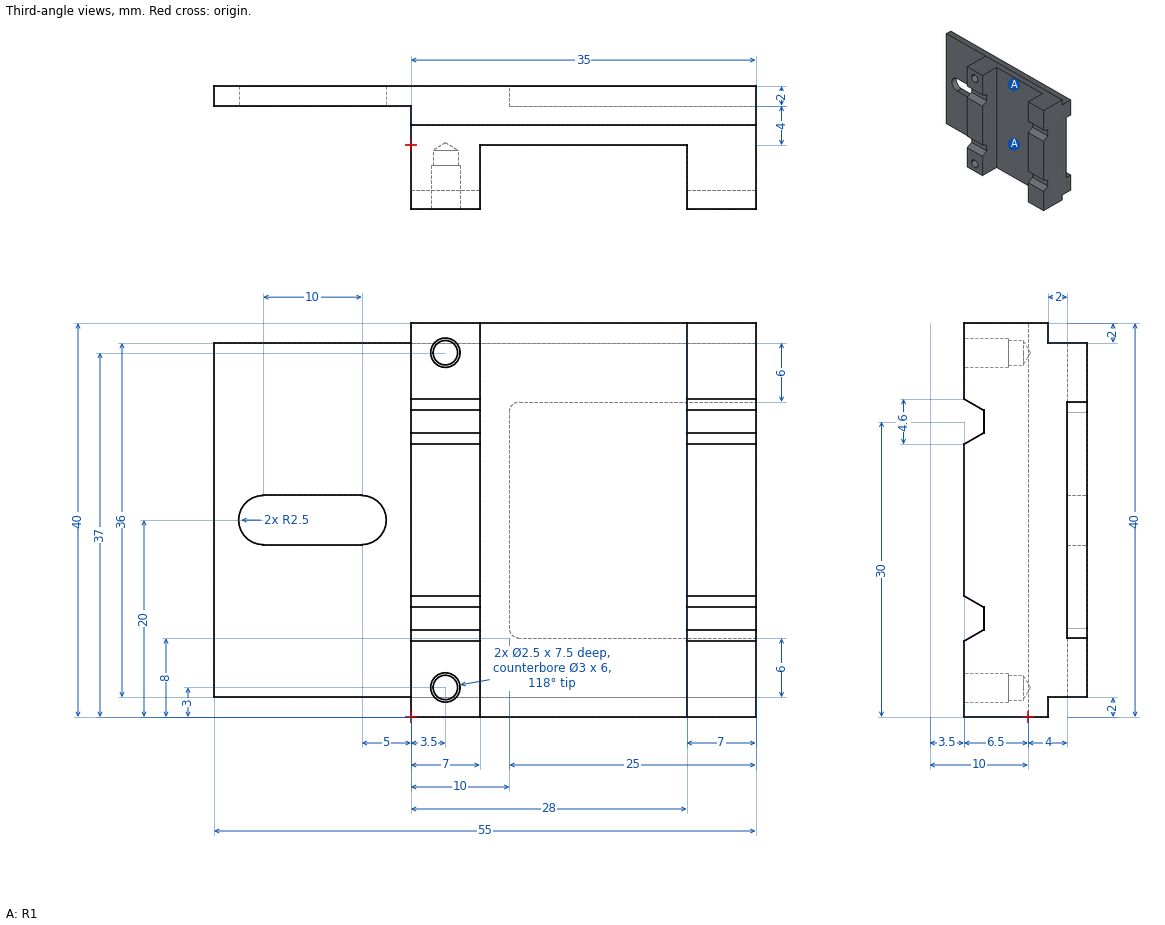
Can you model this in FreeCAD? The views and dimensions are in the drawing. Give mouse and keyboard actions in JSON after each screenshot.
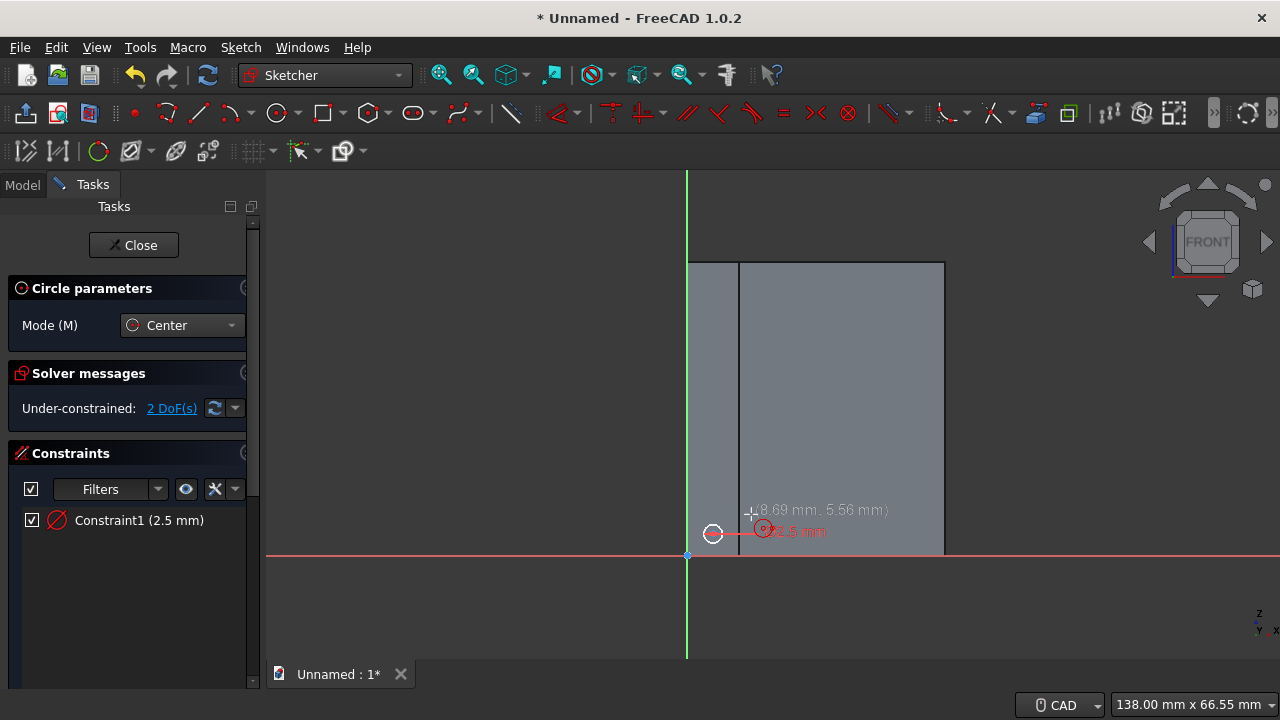
{"action": "scroll", "coordinate": [713, 284], "scroll_direction": "up", "scroll_amount": 5}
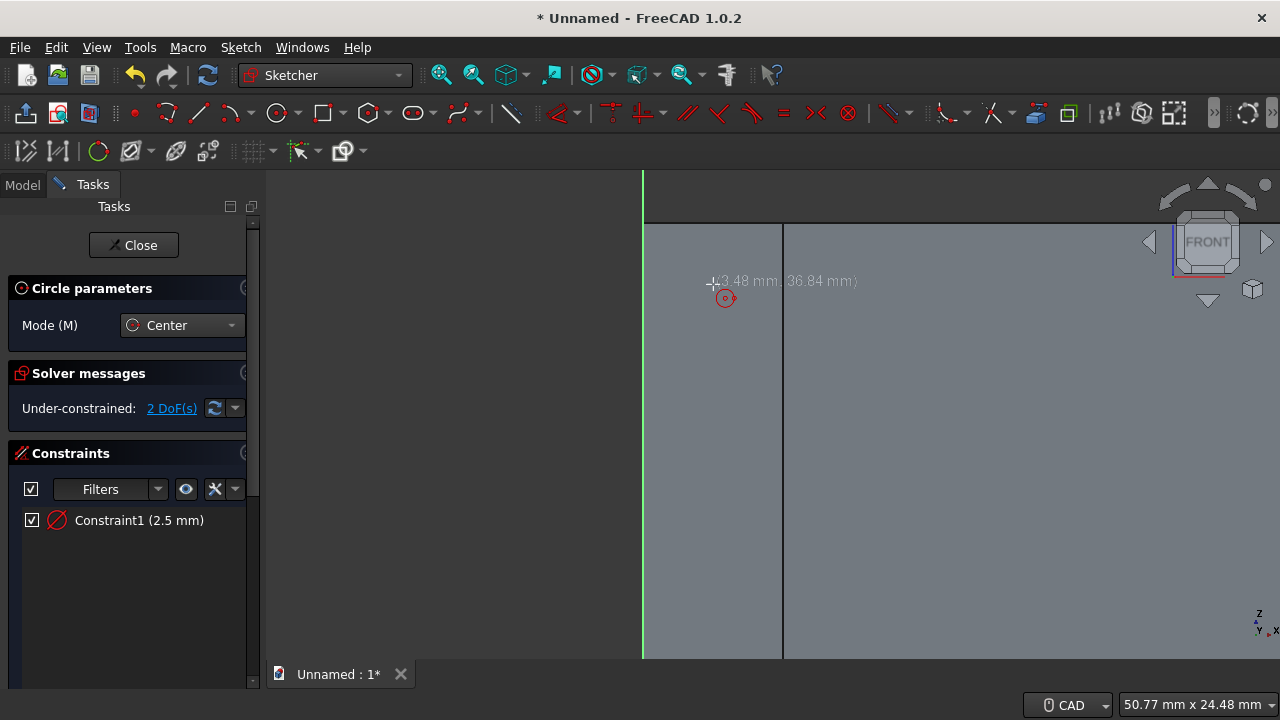
{"action": "left_click", "coordinate": [713, 283]}
{"action": "mouse_move", "coordinate": [730, 265]}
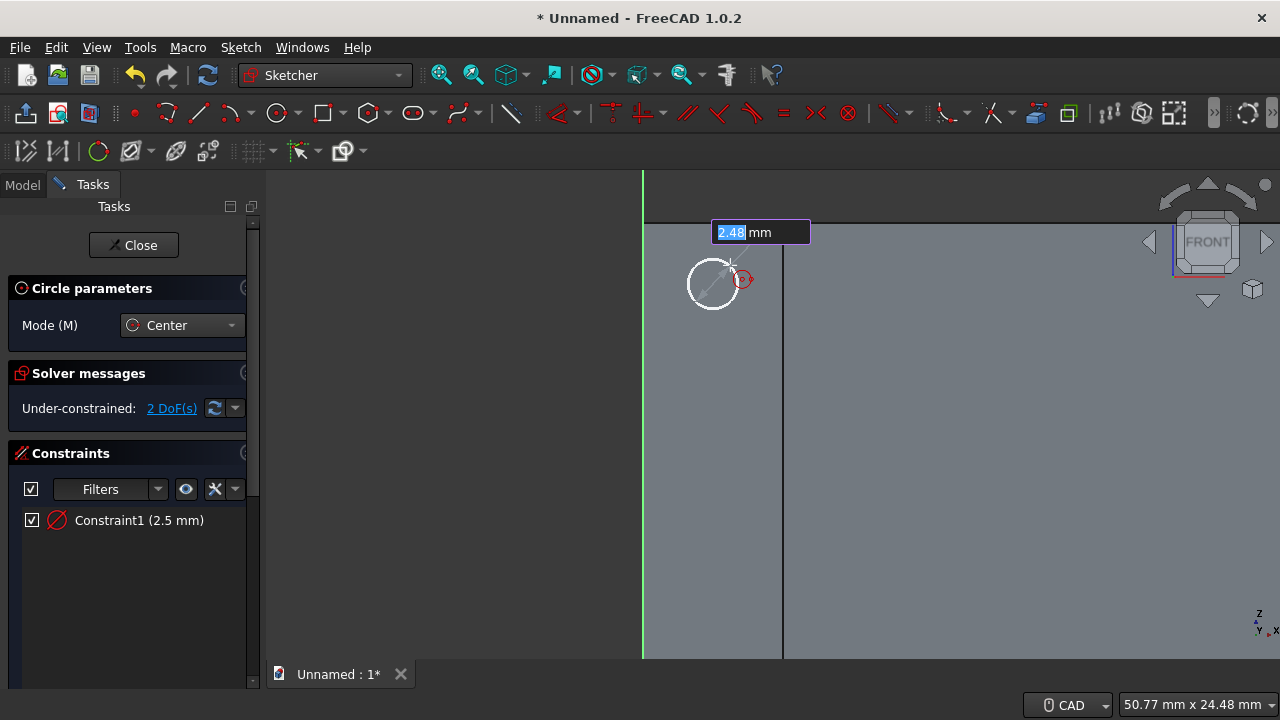
{"action": "type", "text": "2.5"}
{"action": "key", "text": "Return"}
{"action": "key", "text": "Escape"}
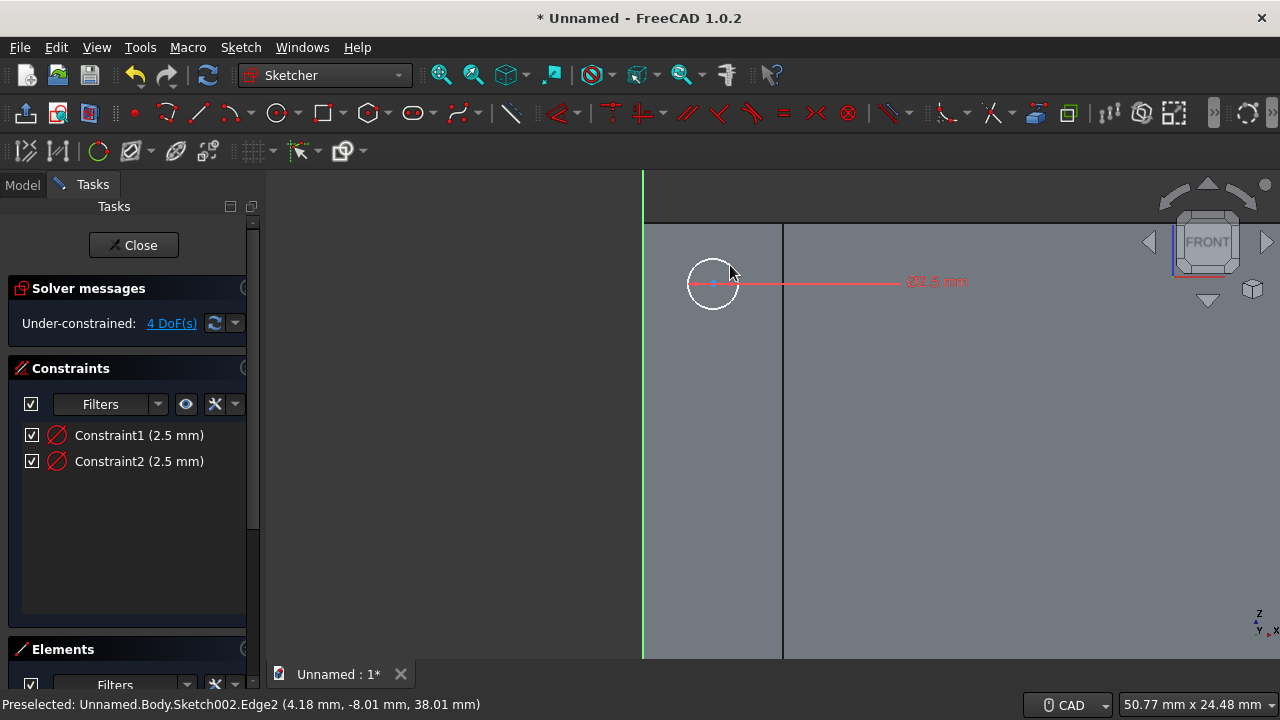
{"action": "scroll", "coordinate": [713, 283], "scroll_direction": "down", "scroll_amount": 5}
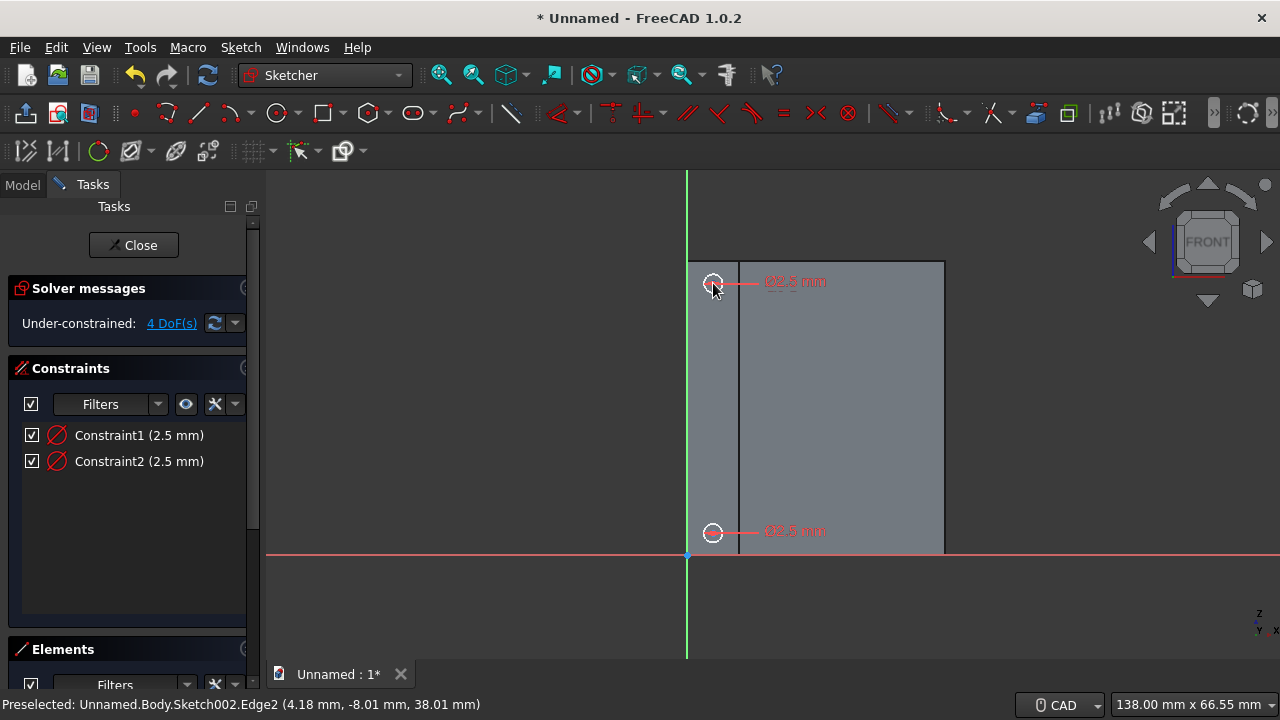
{"action": "left_click", "coordinate": [713, 533]}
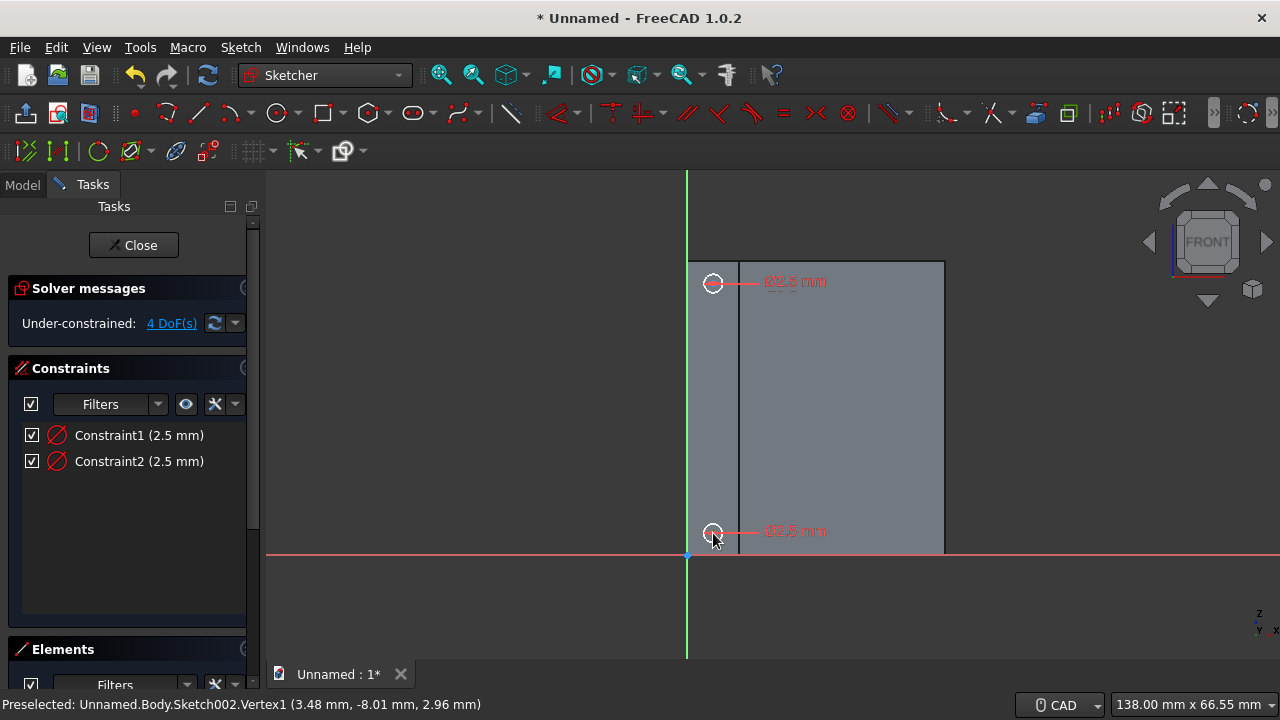
{"action": "left_click", "coordinate": [713, 284]}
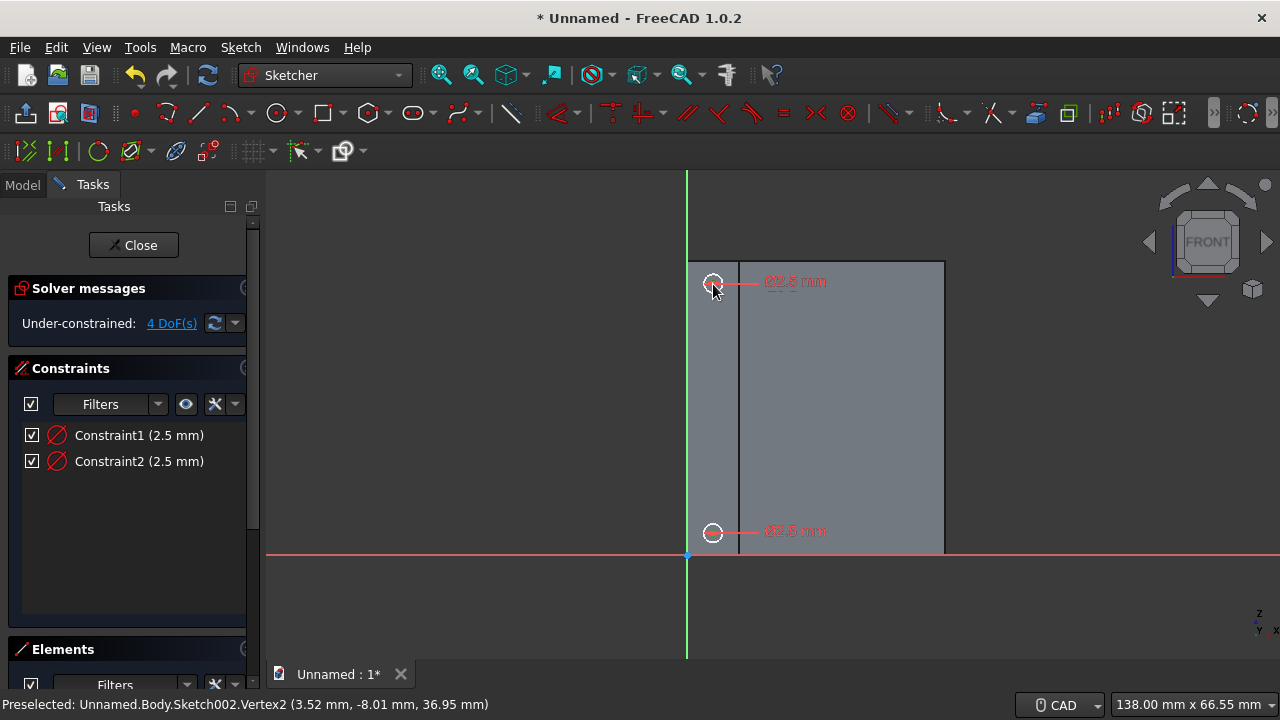
{"action": "key", "text": "v"}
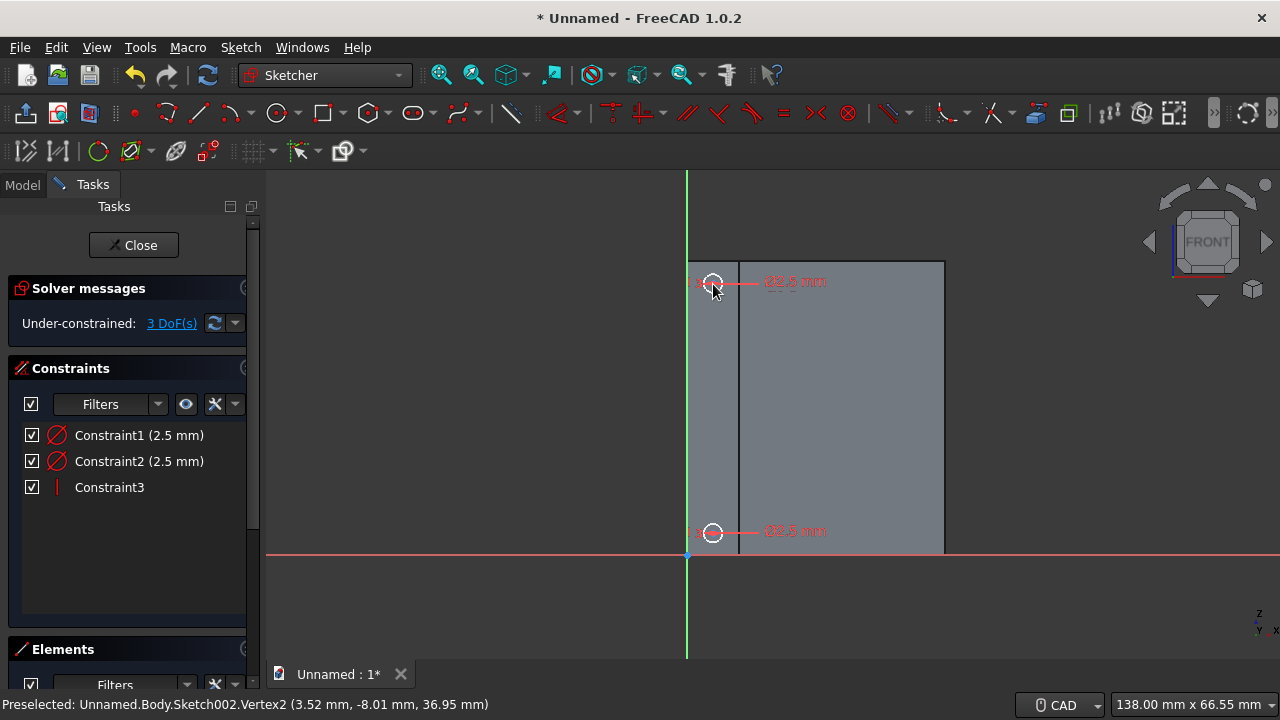
{"action": "scroll", "coordinate": [713, 533], "scroll_direction": "up", "scroll_amount": 3}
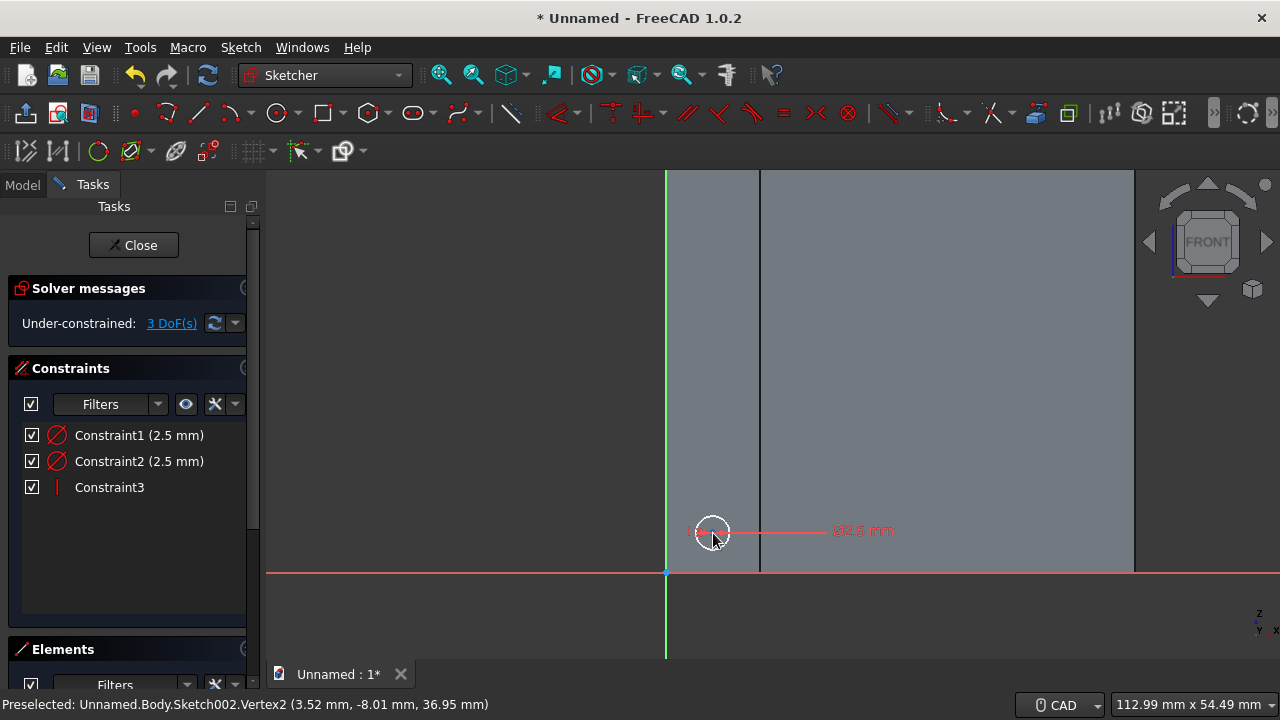
{"action": "left_click", "coordinate": [713, 533]}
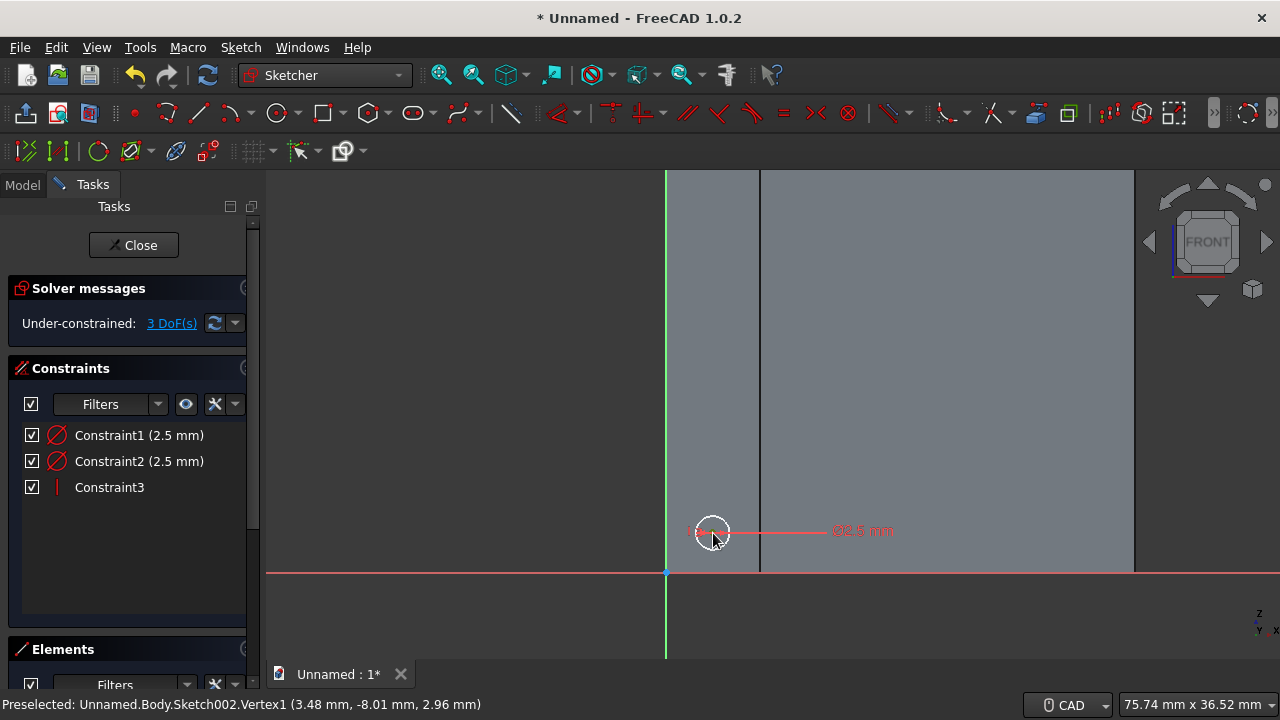
{"action": "left_click", "coordinate": [580, 114]}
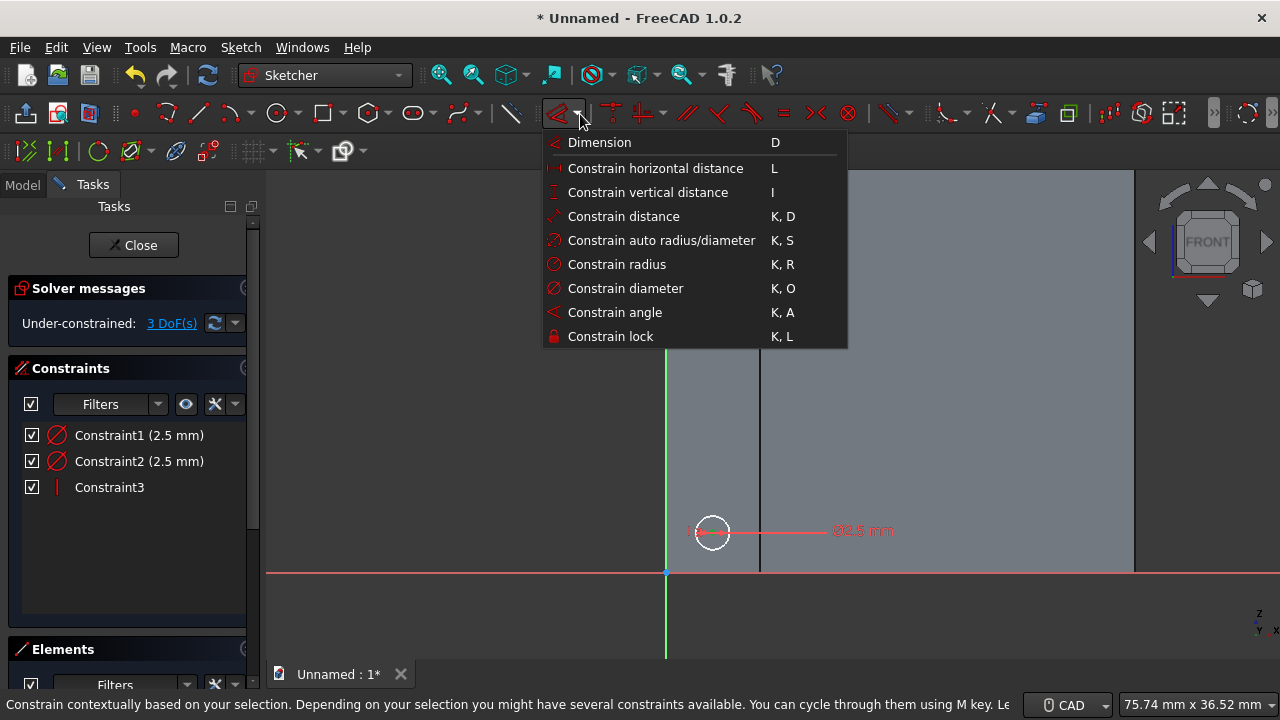
{"action": "left_click", "coordinate": [695, 192]}